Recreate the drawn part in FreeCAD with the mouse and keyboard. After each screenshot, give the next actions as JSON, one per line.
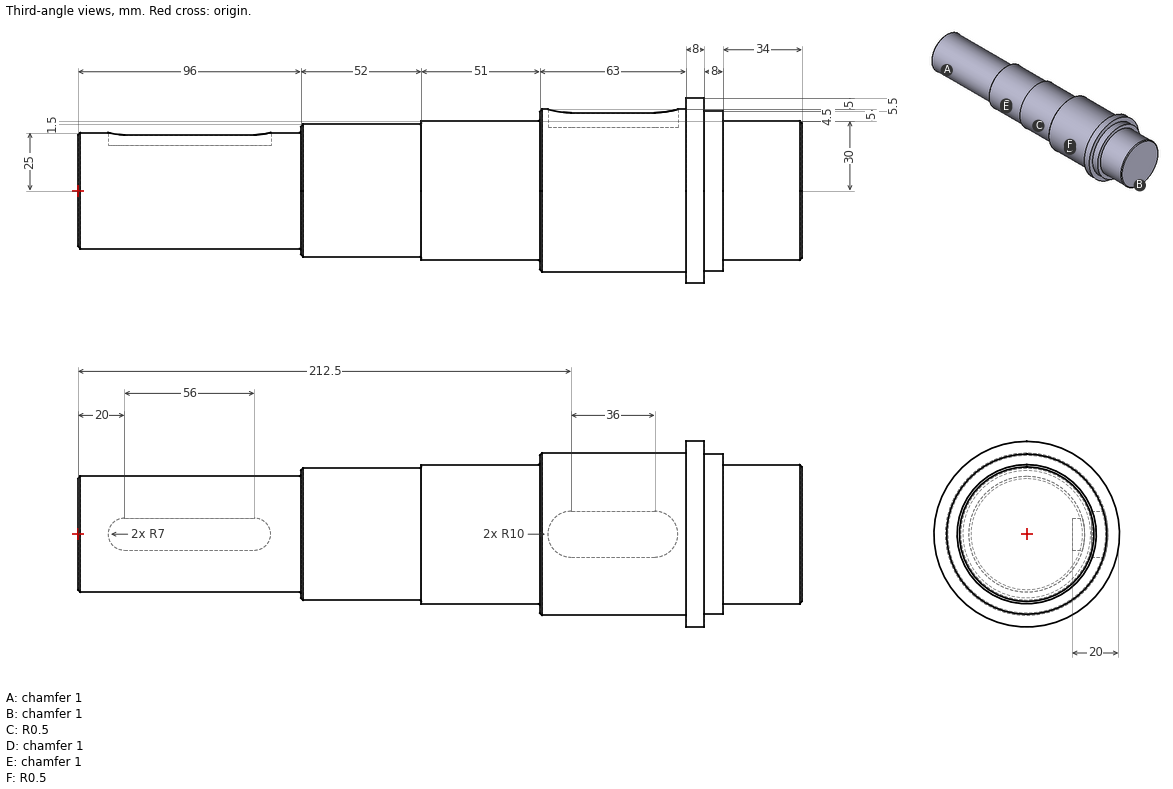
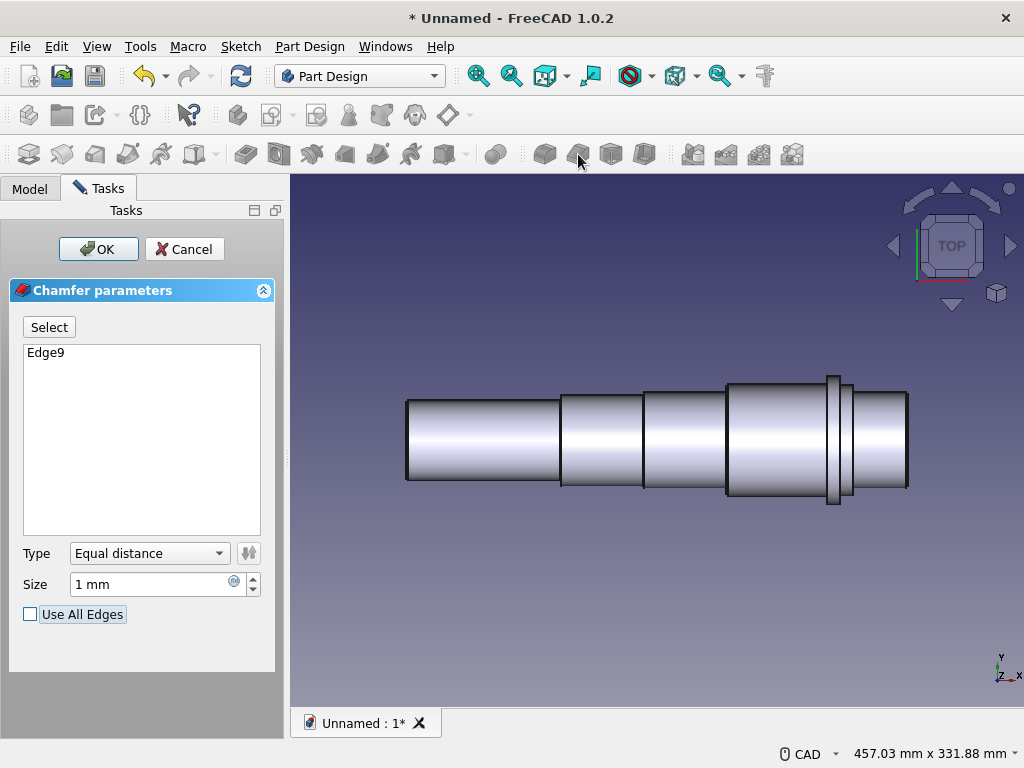
{"action": "left_click", "coordinate": [99, 249]}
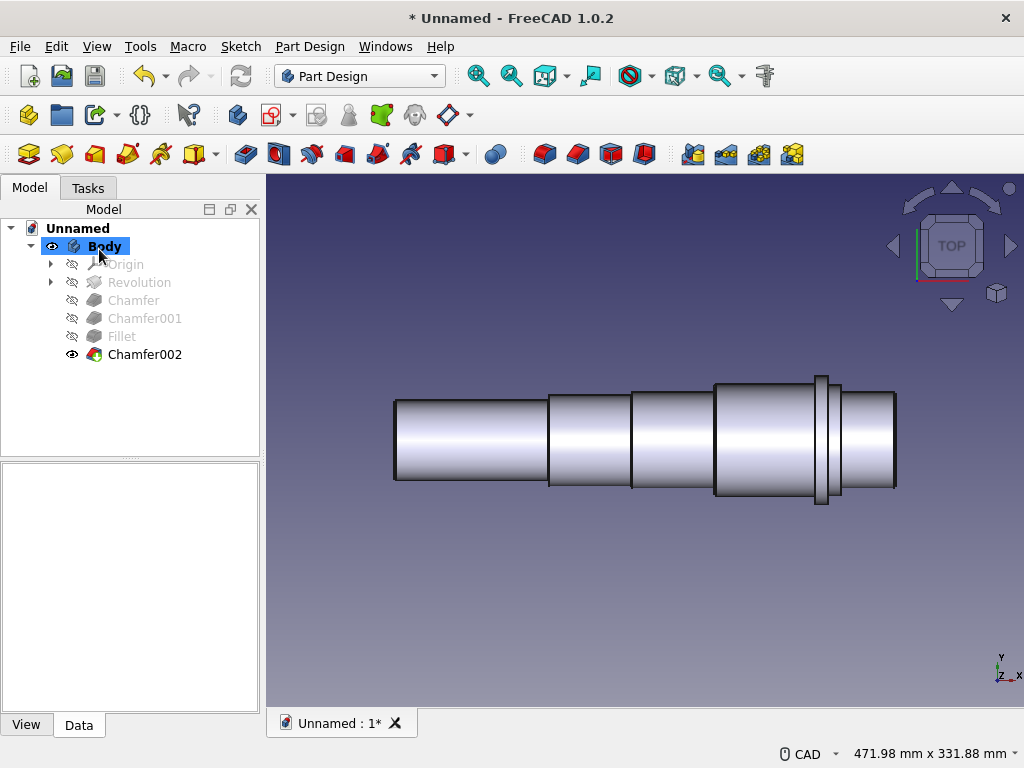
{"action": "left_click", "coordinate": [549, 477]}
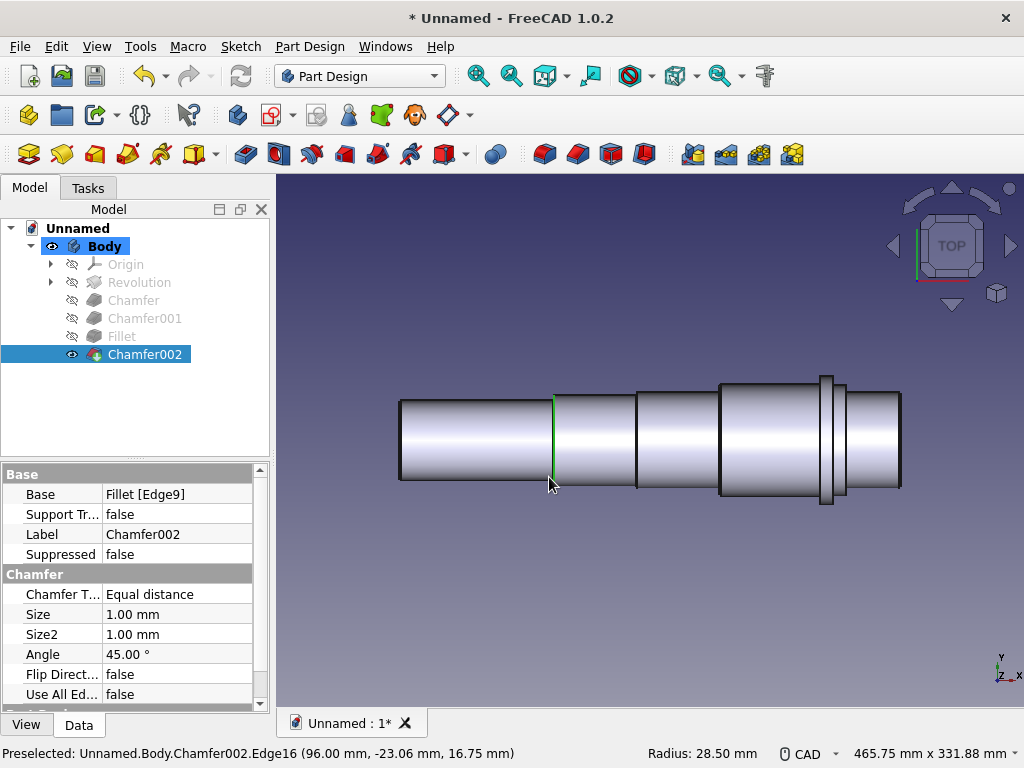
{"action": "left_click", "coordinate": [578, 154]}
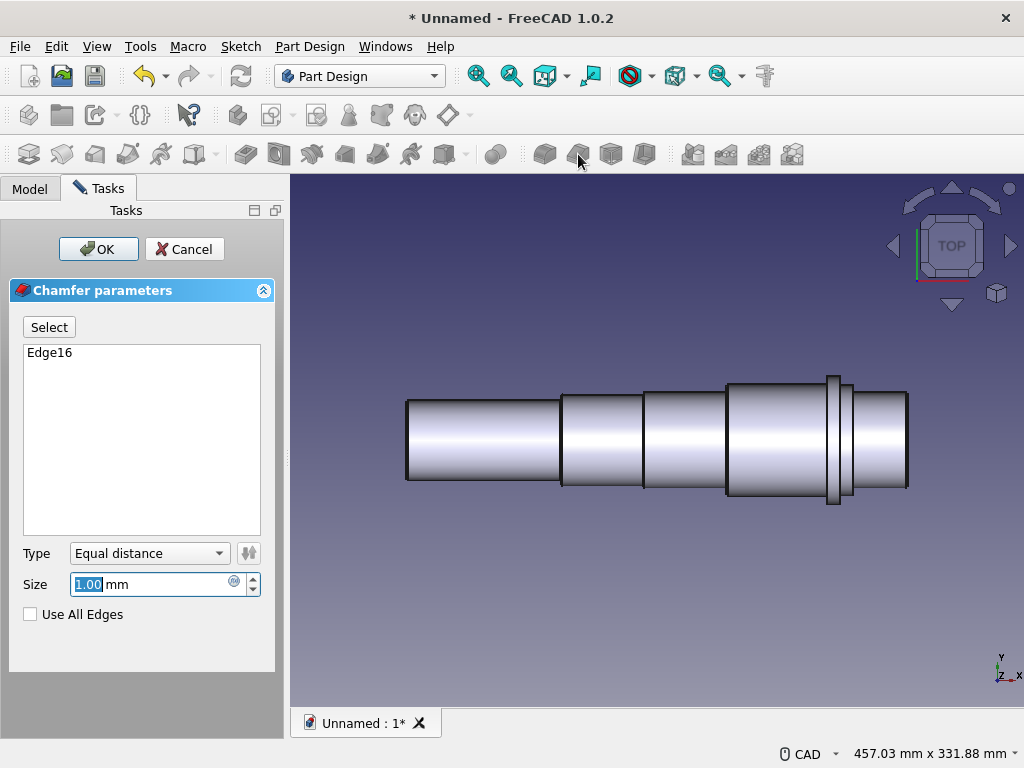
{"action": "type", "text": "1"}
{"action": "key", "text": "Tab"}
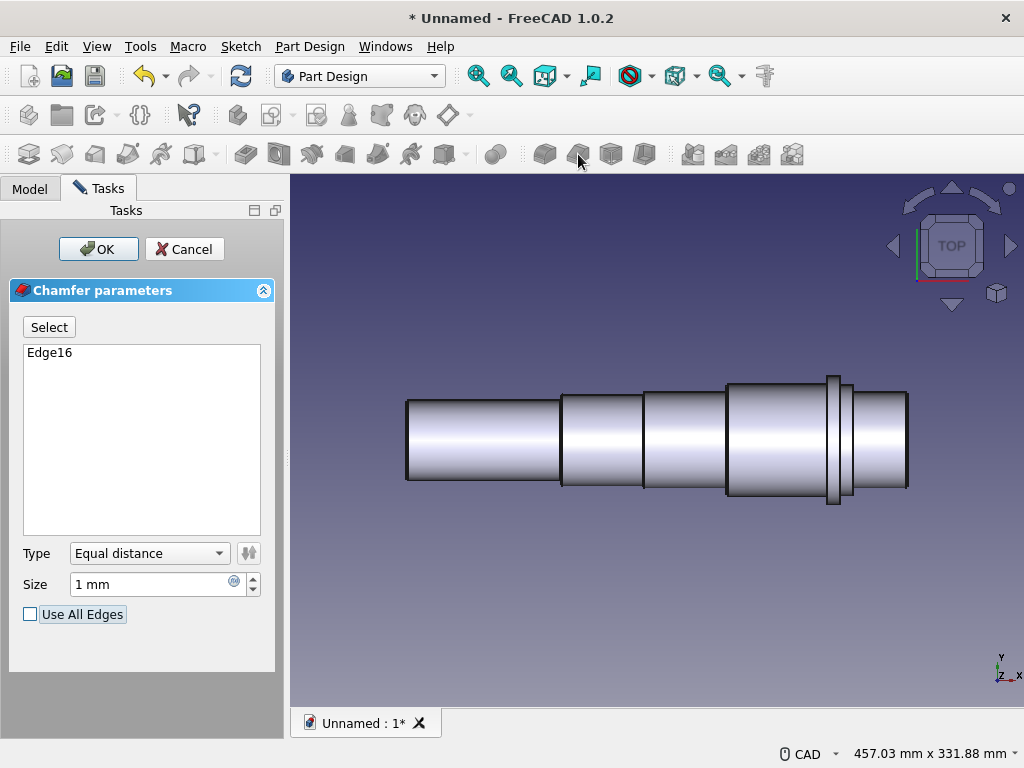
{"action": "left_click", "coordinate": [99, 249]}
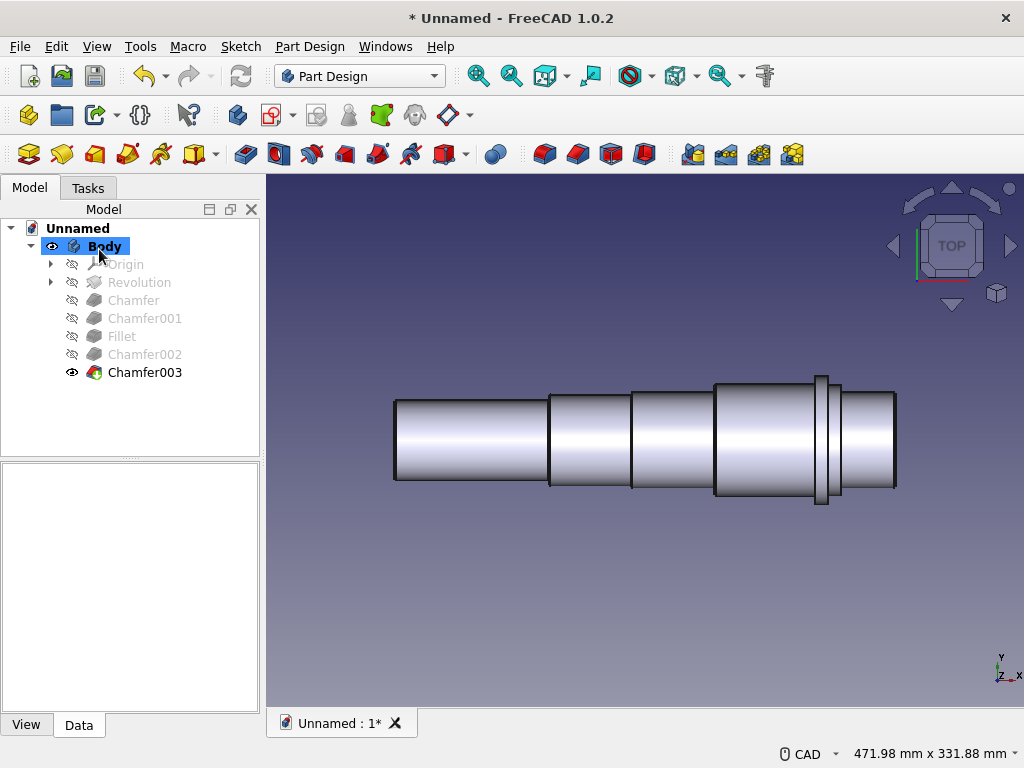
{"action": "key", "text": "0"}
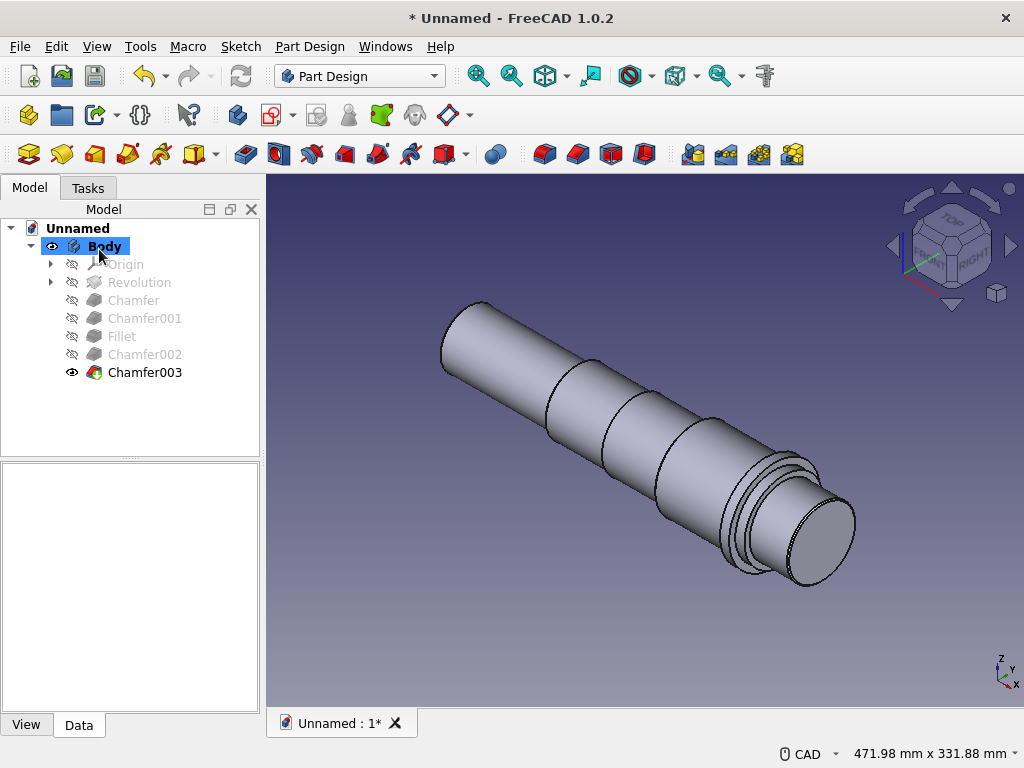
{"action": "key", "text": "2"}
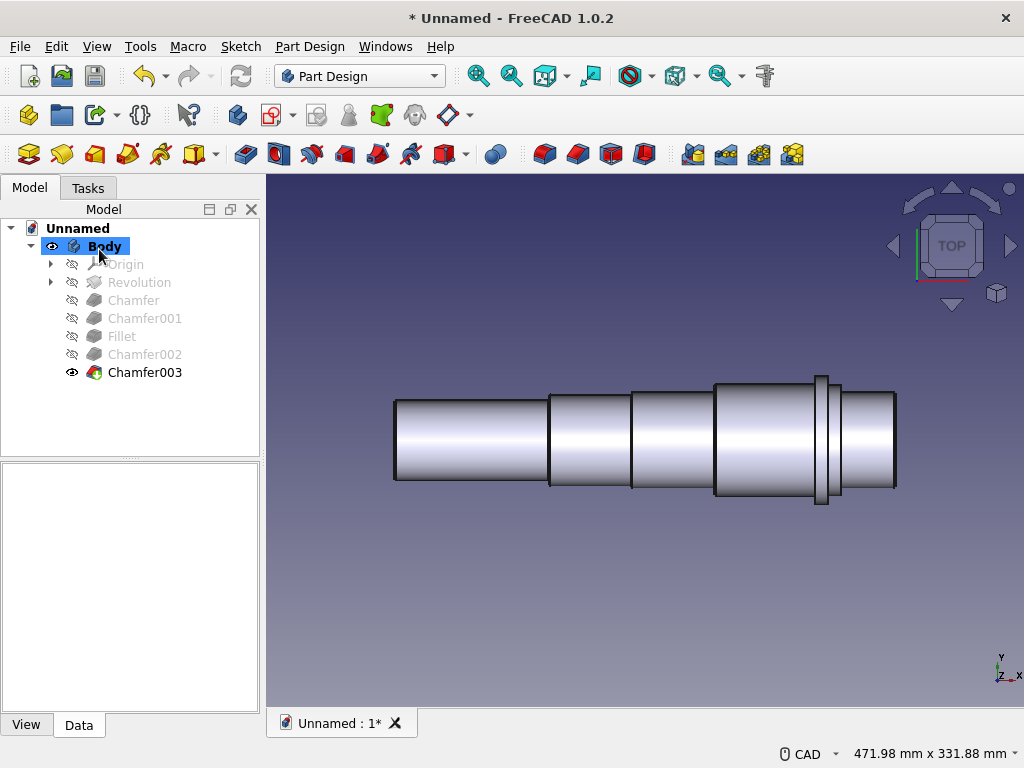
{"action": "key", "text": "1"}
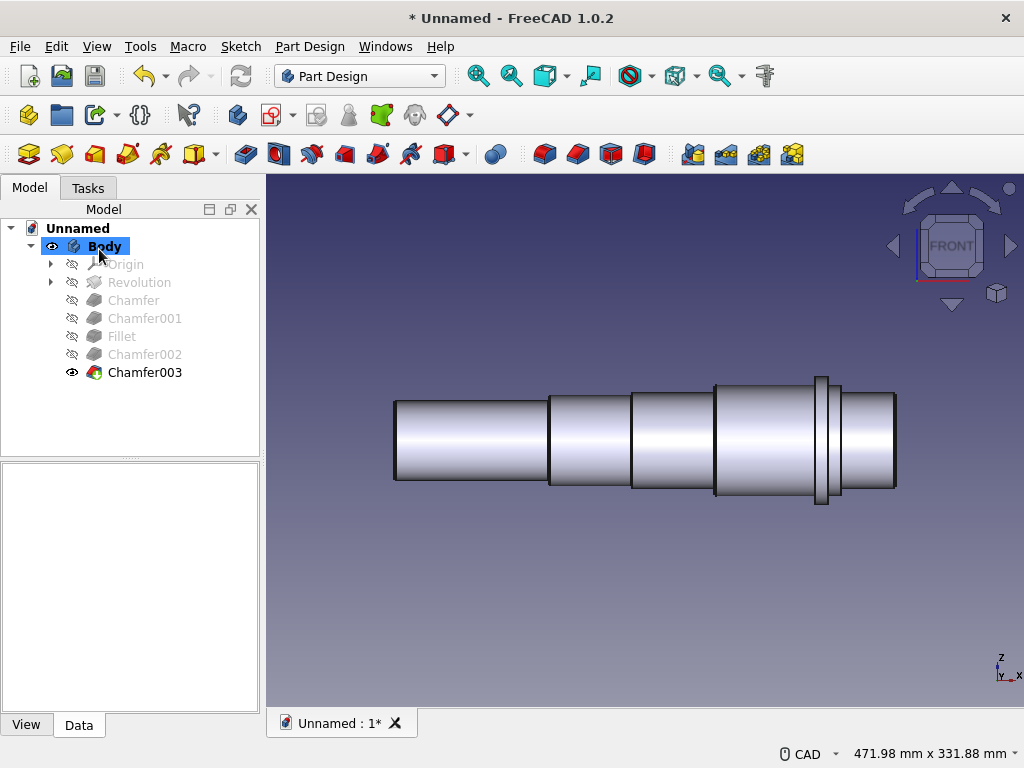
{"action": "key", "text": "3"}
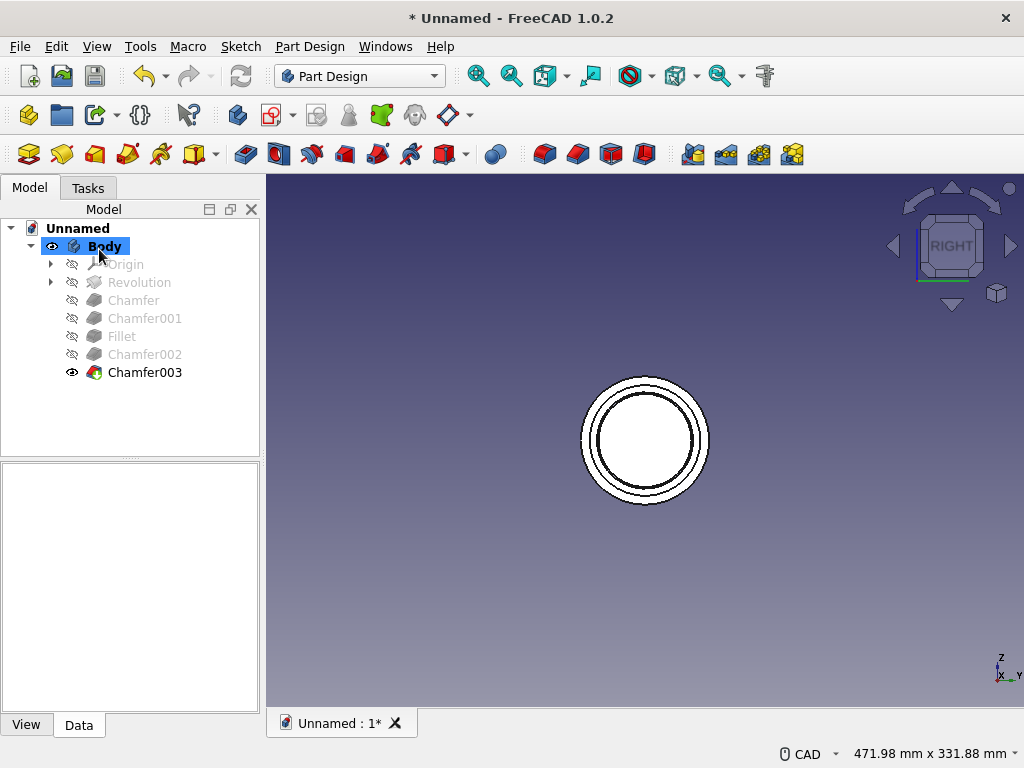
{"action": "key", "text": "v f"}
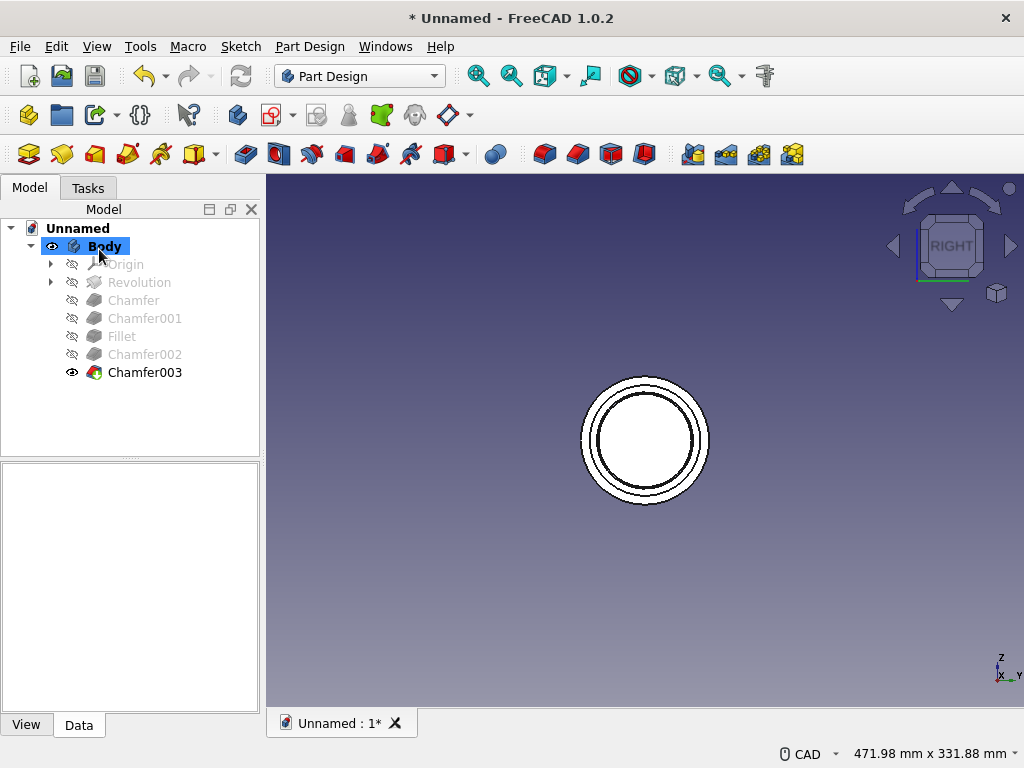
{"action": "key", "text": "5"}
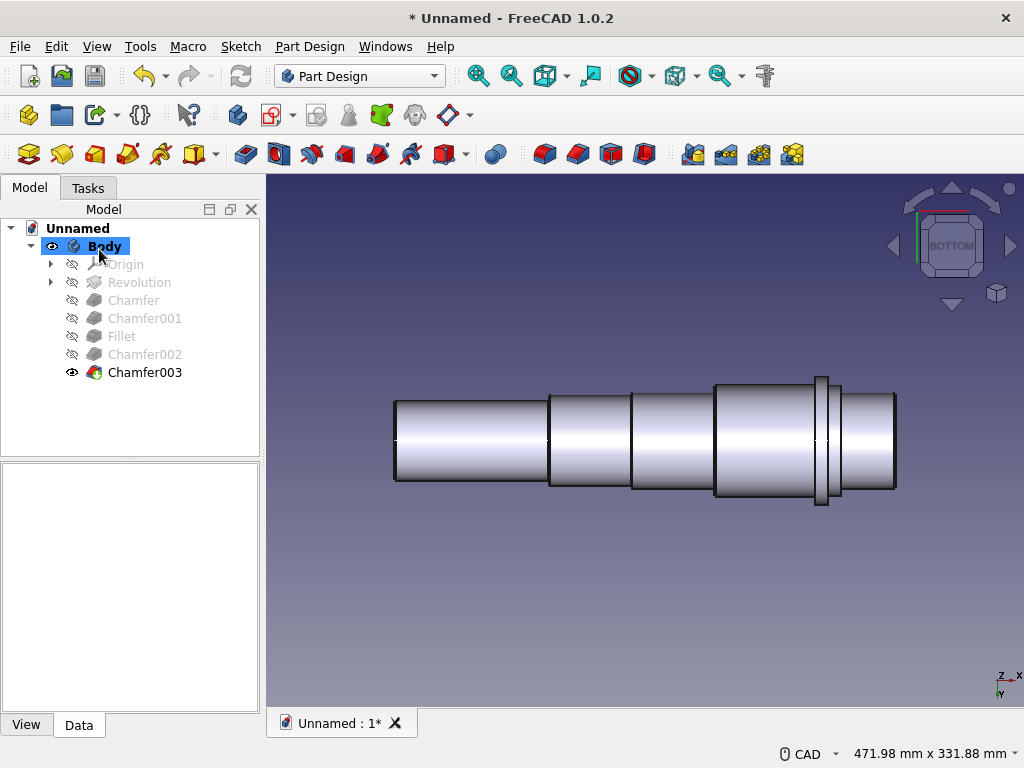
{"action": "key", "text": "4"}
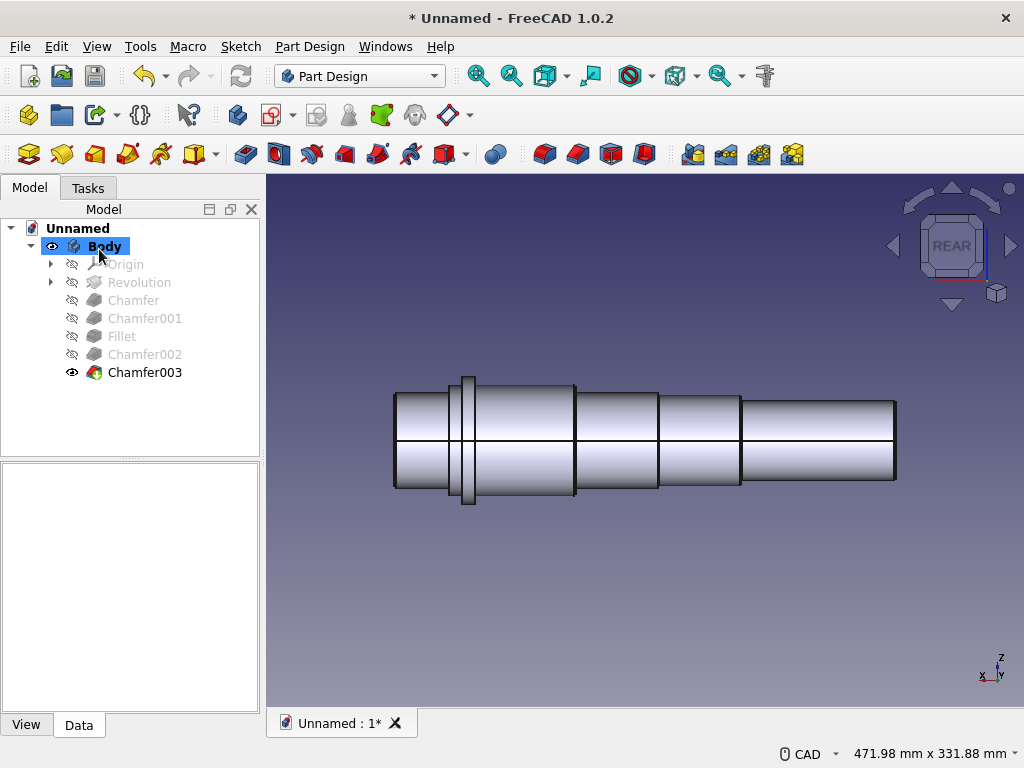
{"action": "key", "text": "6"}